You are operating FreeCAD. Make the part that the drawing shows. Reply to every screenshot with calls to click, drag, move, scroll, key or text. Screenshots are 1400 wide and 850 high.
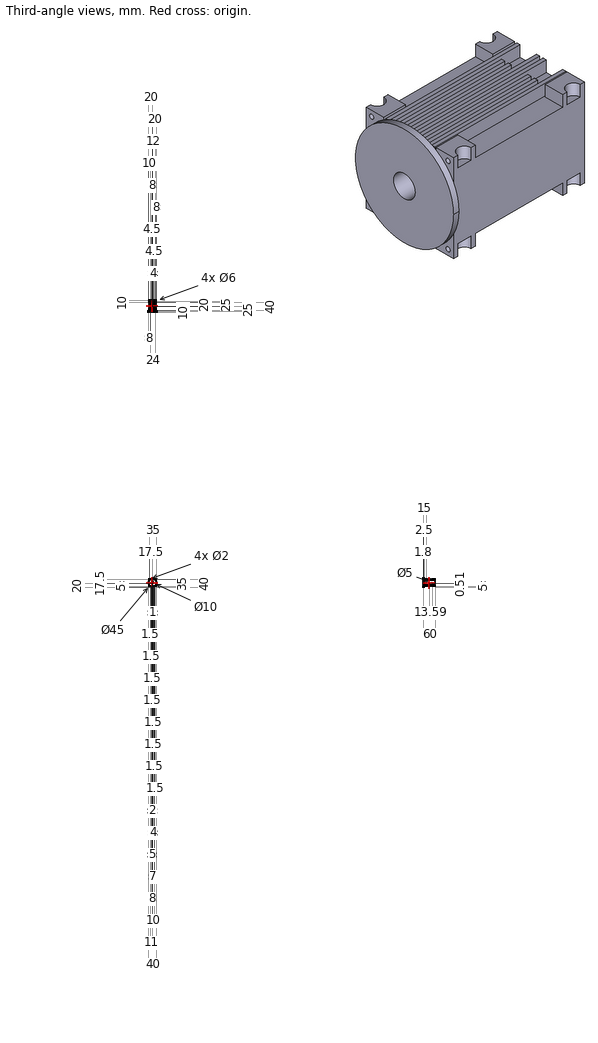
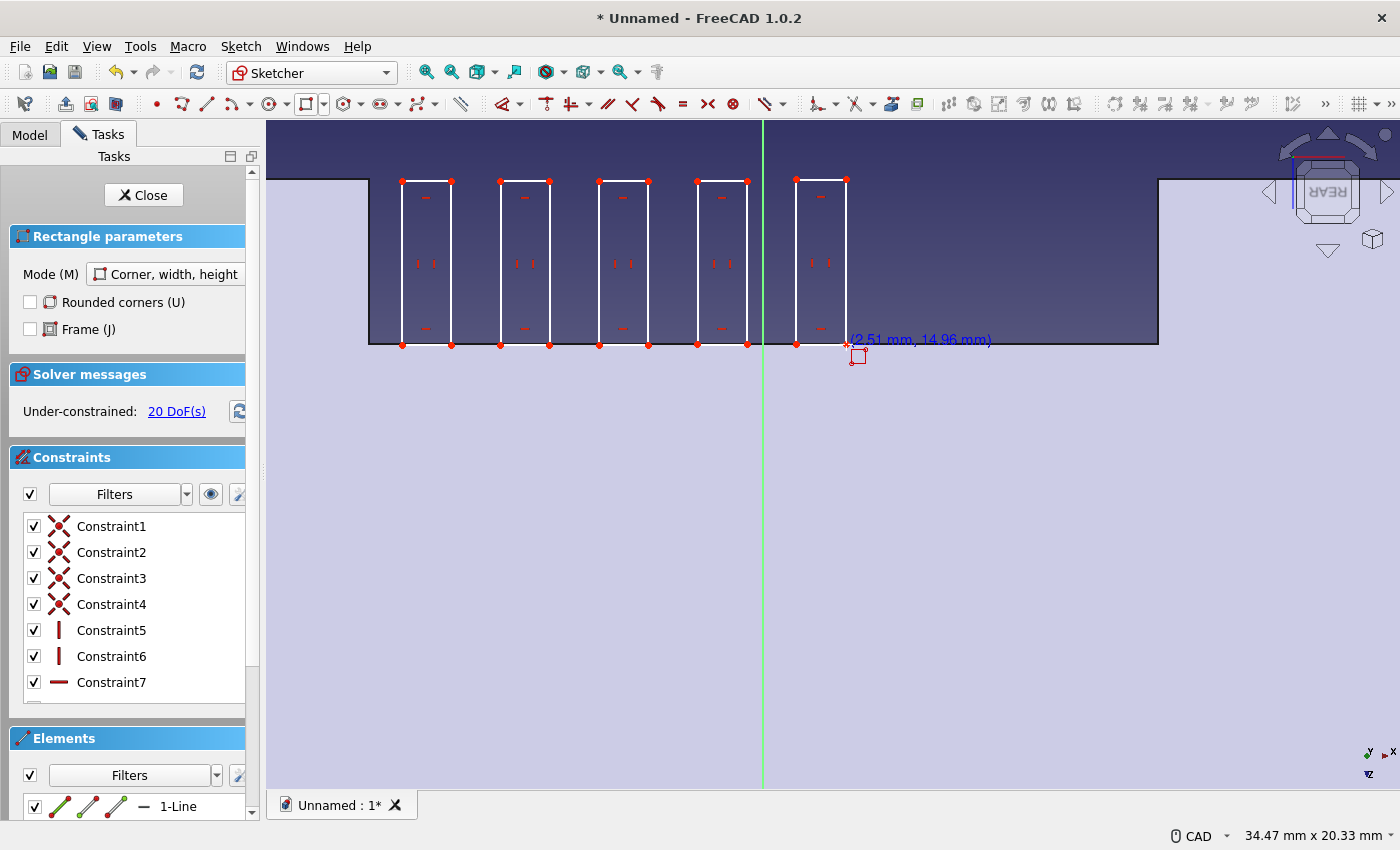
click(895, 179)
click(944, 344)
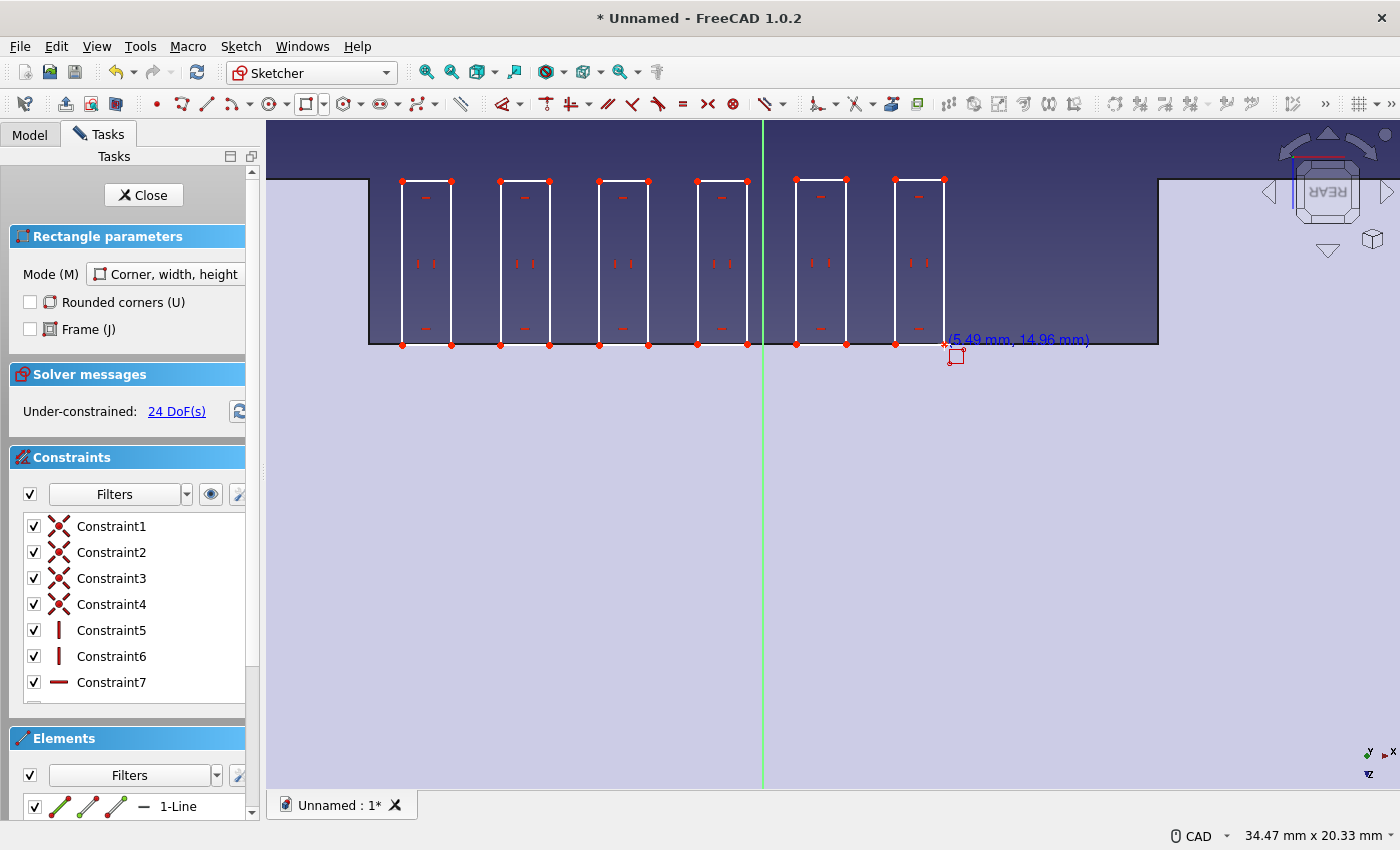
click(994, 179)
click(1043, 344)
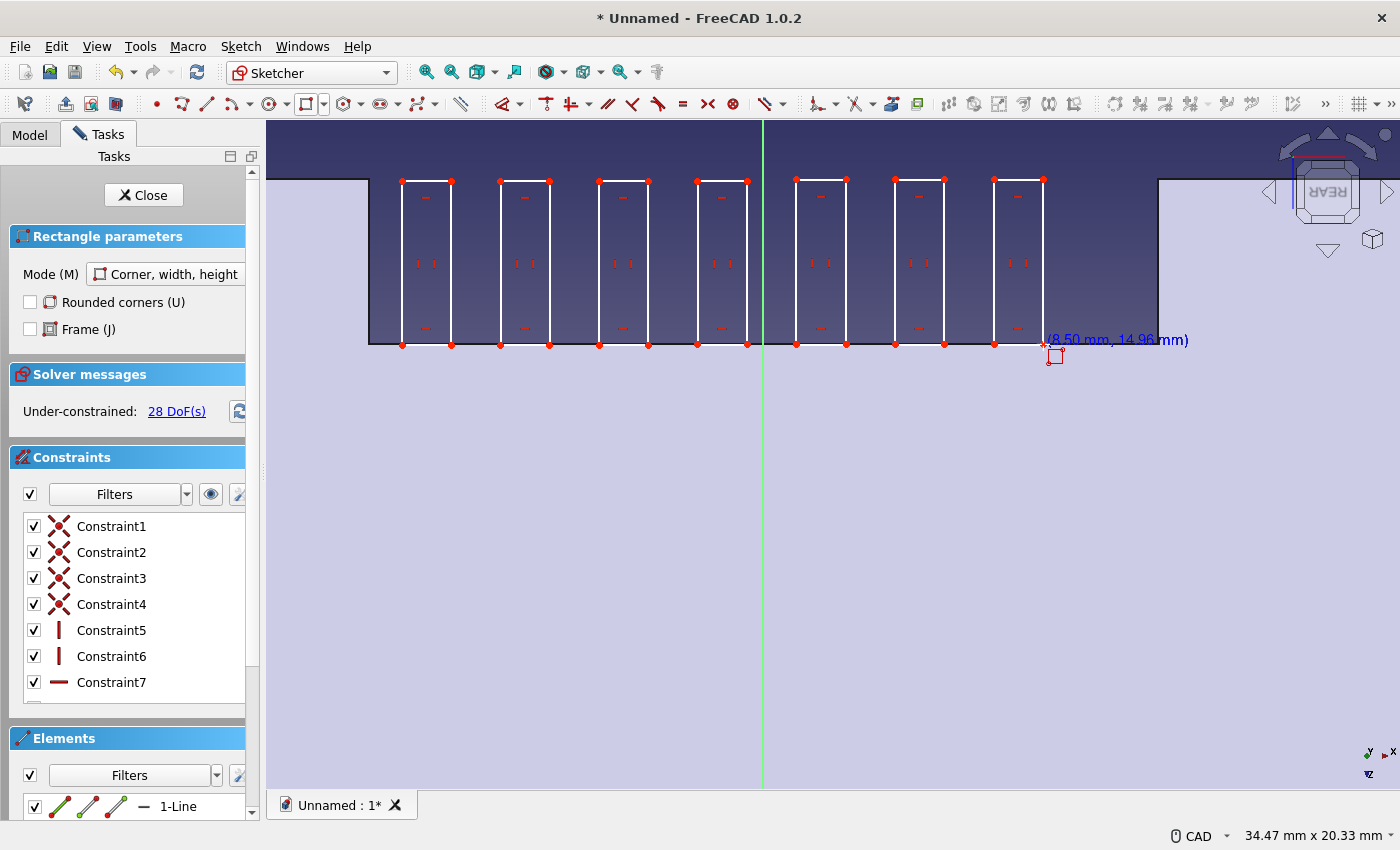
click(1092, 179)
click(1142, 344)
key(Escape)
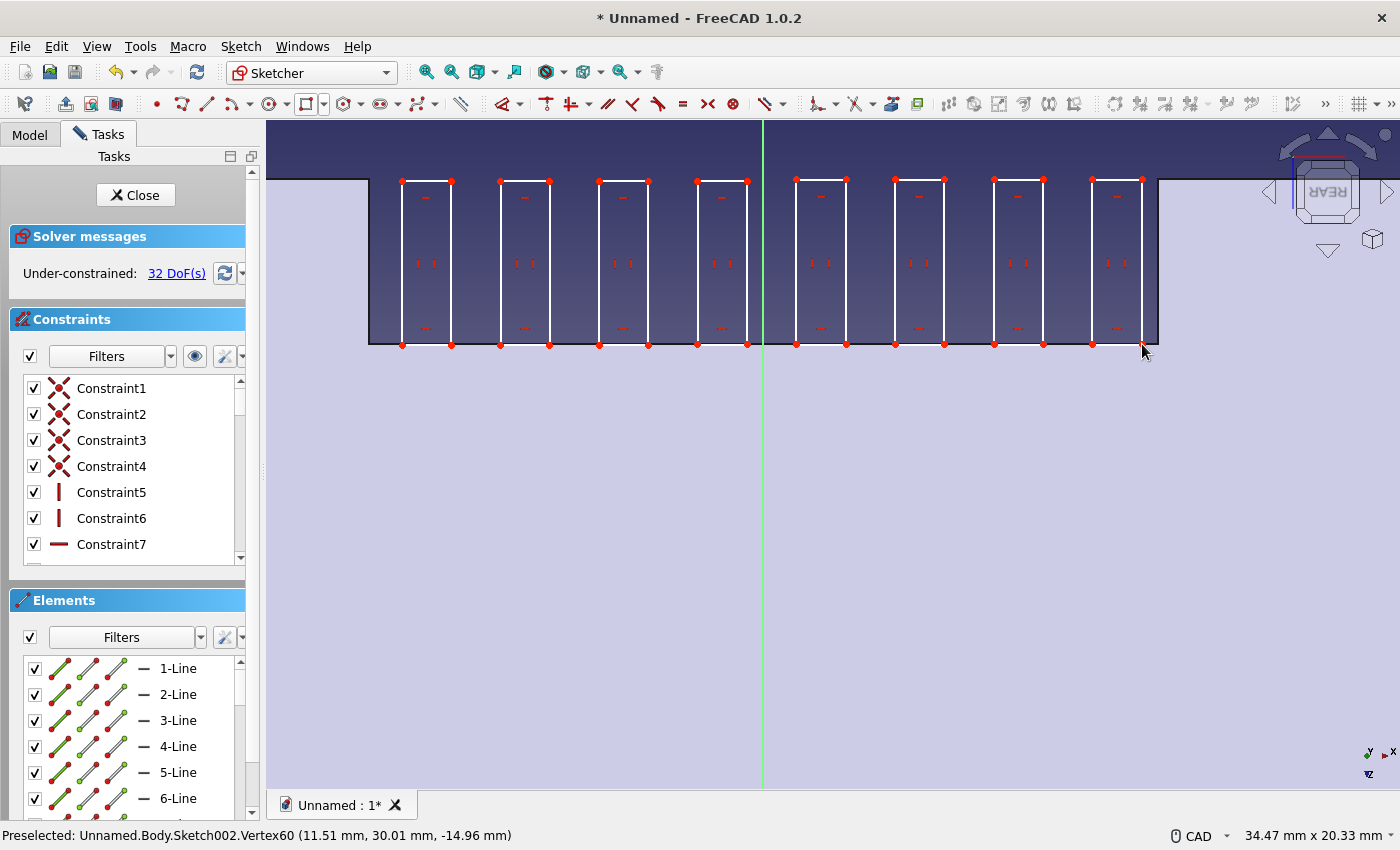
key(d)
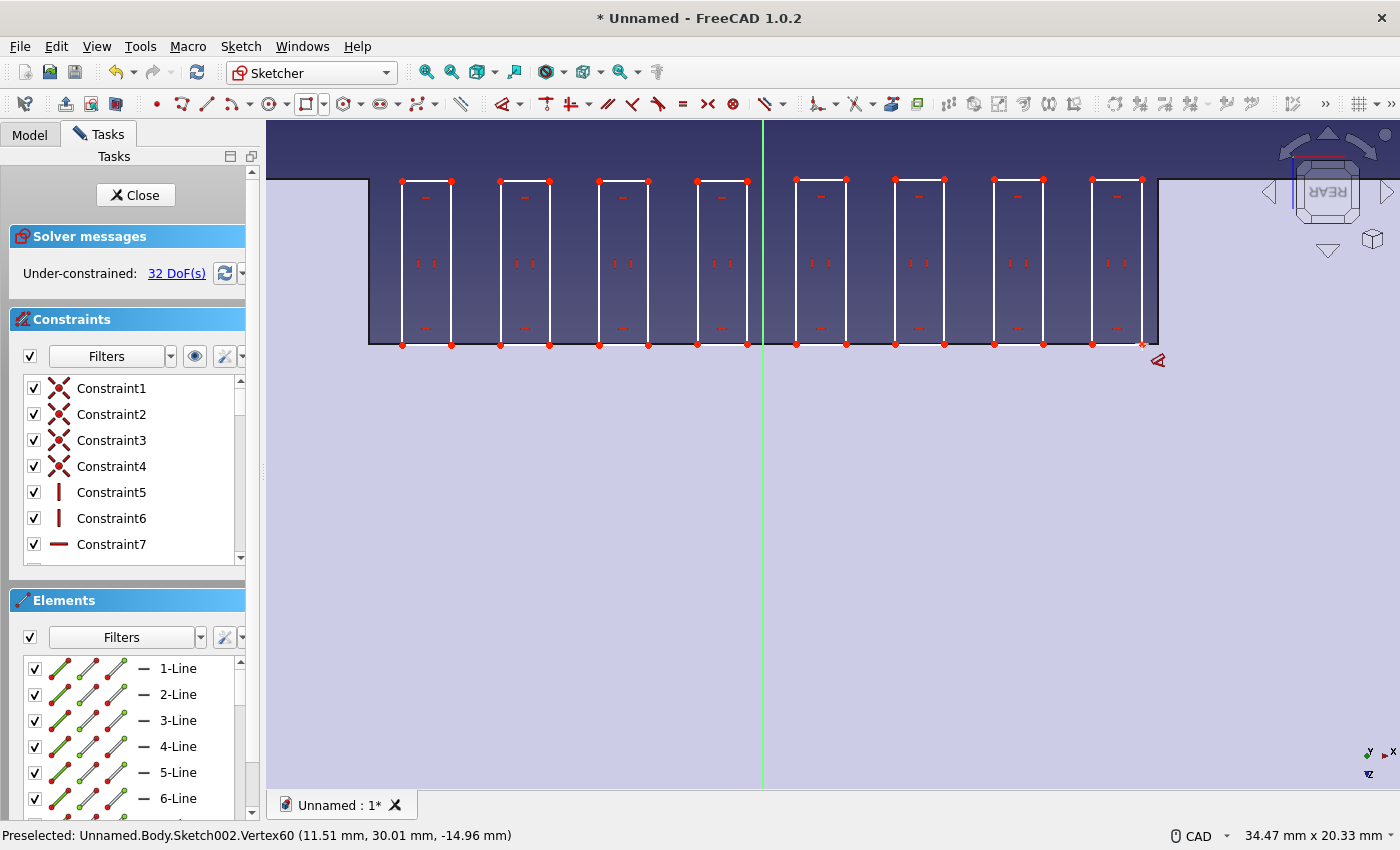
click(402, 230)
click(368, 263)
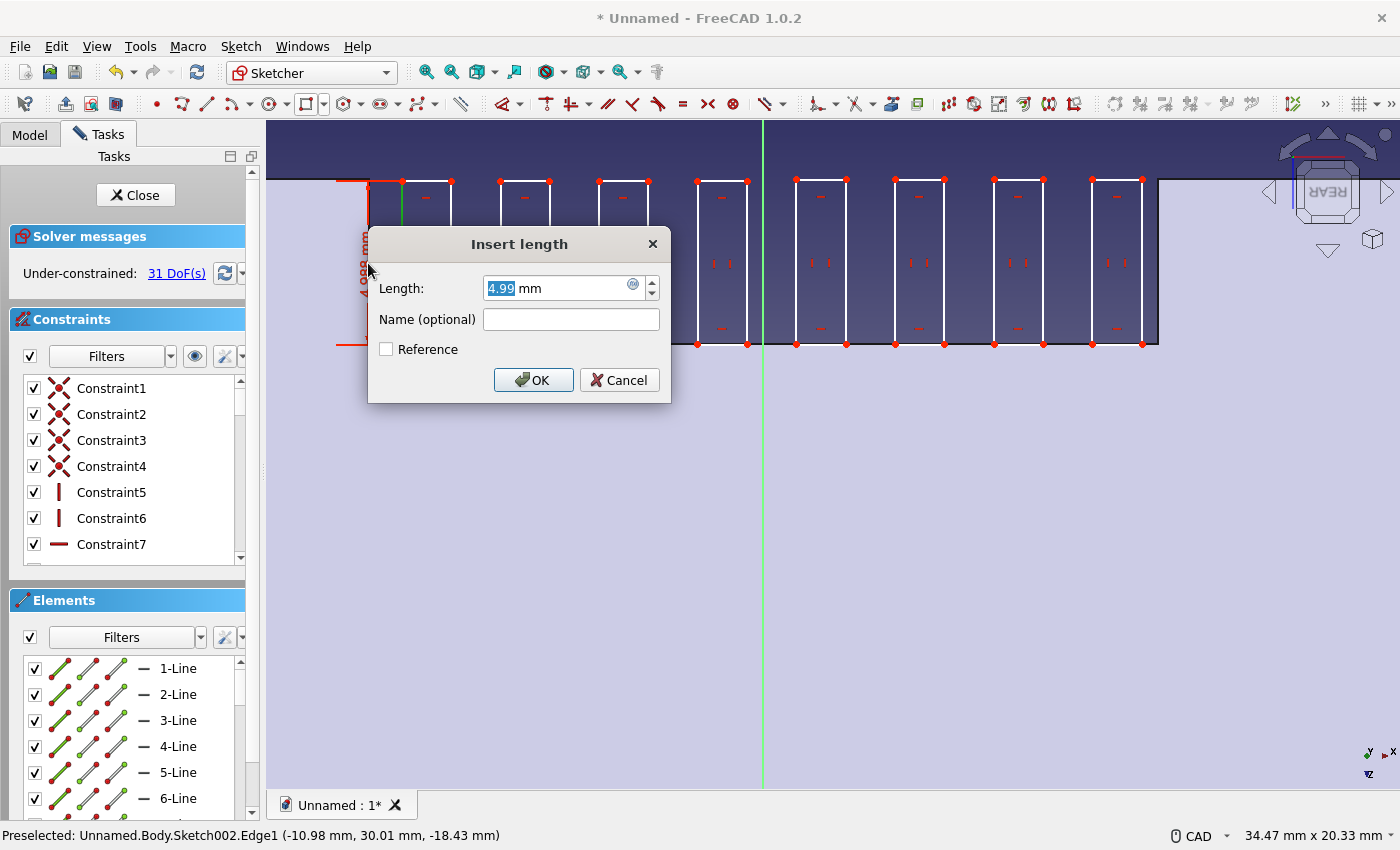
text(5)
key(Return)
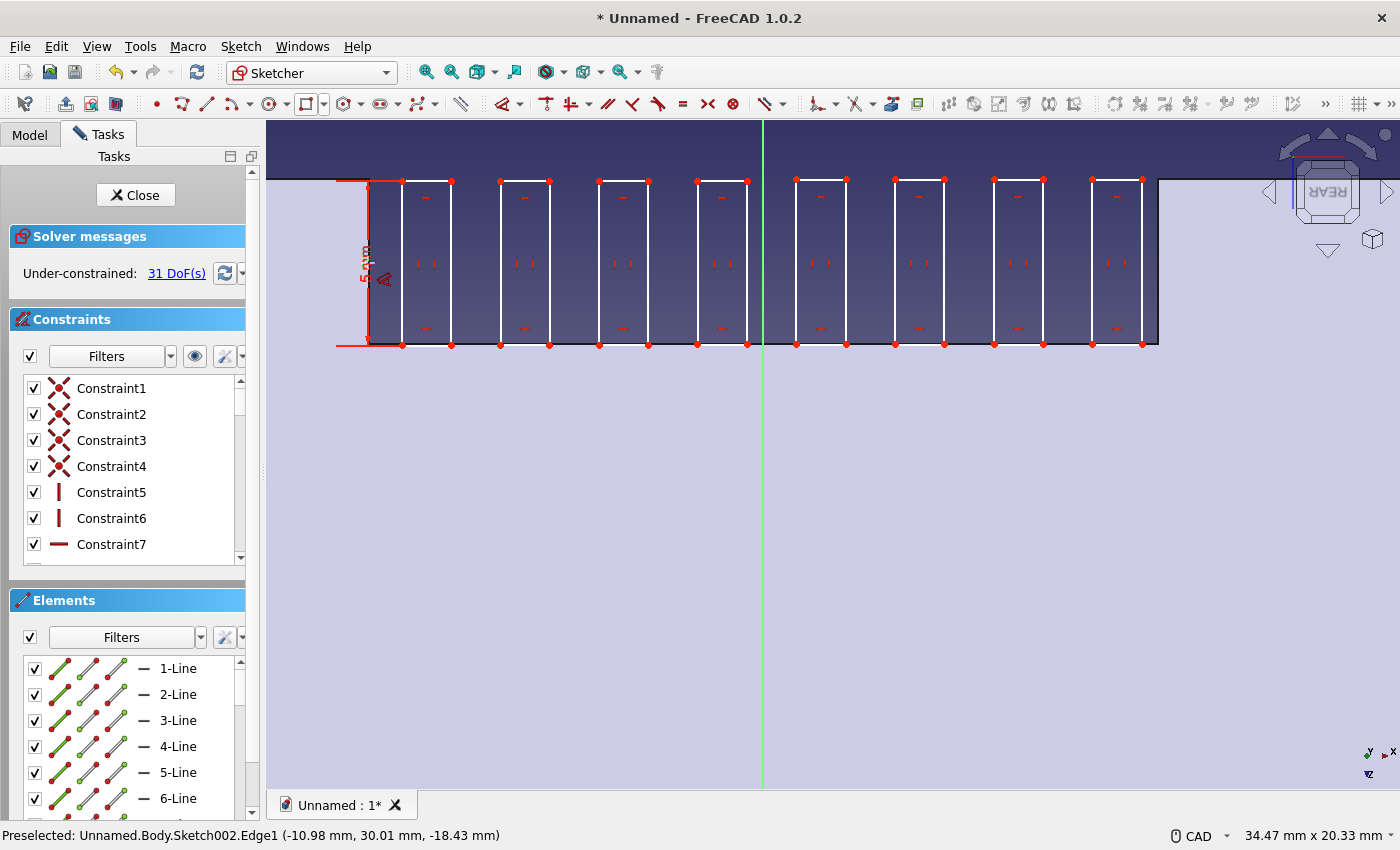
click(501, 230)
click(467, 263)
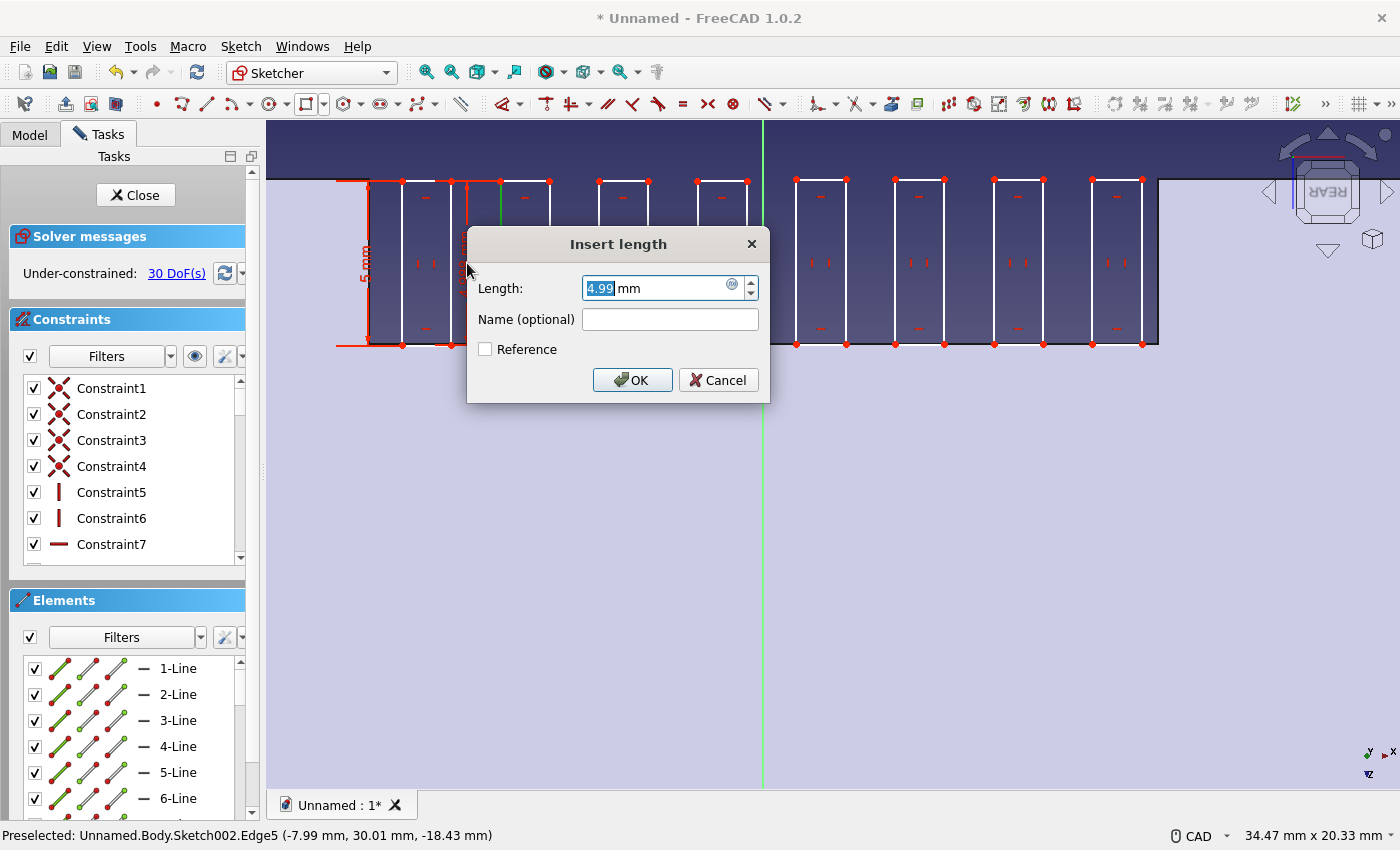
text(5)
key(Return)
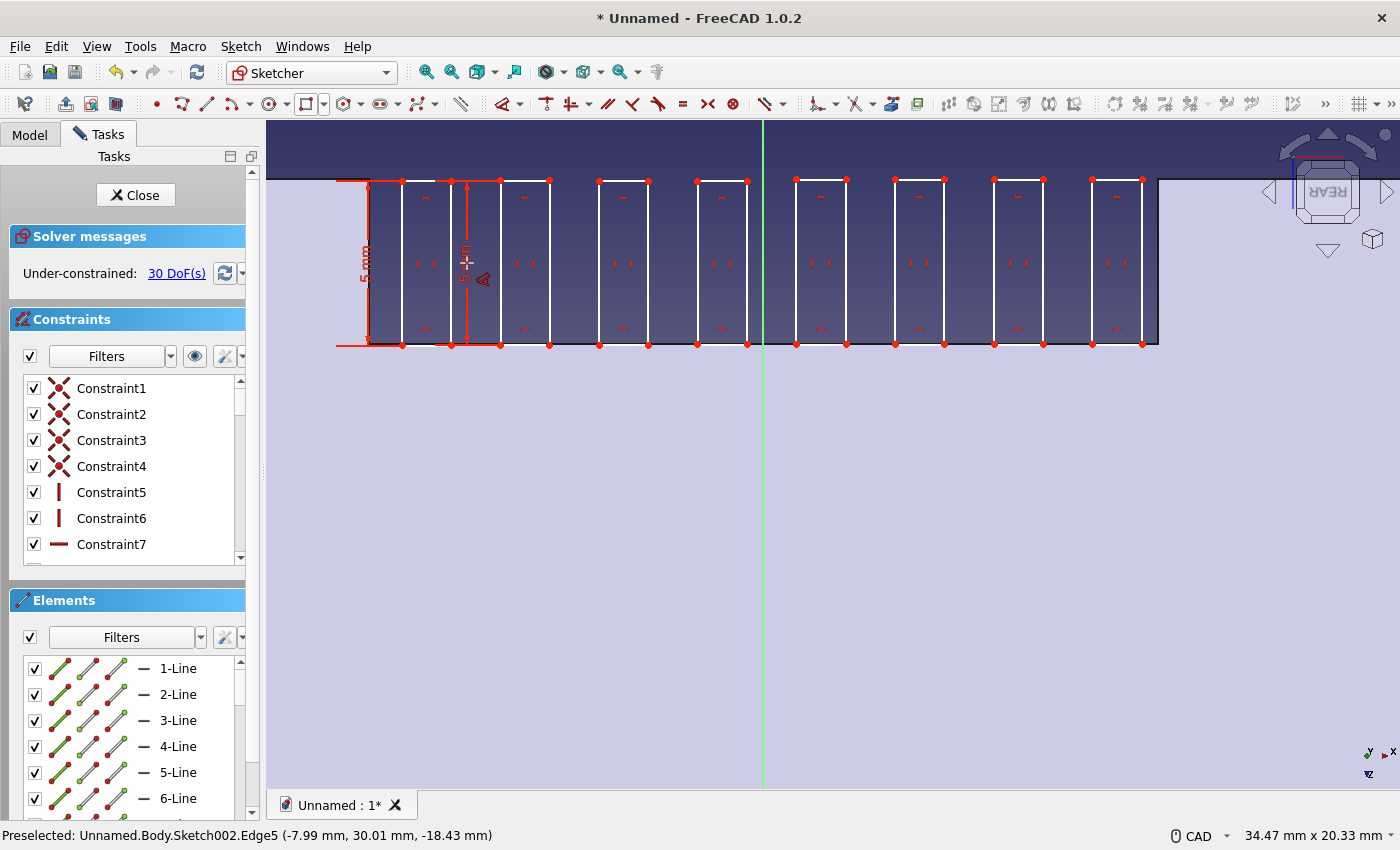
click(599, 230)
click(565, 263)